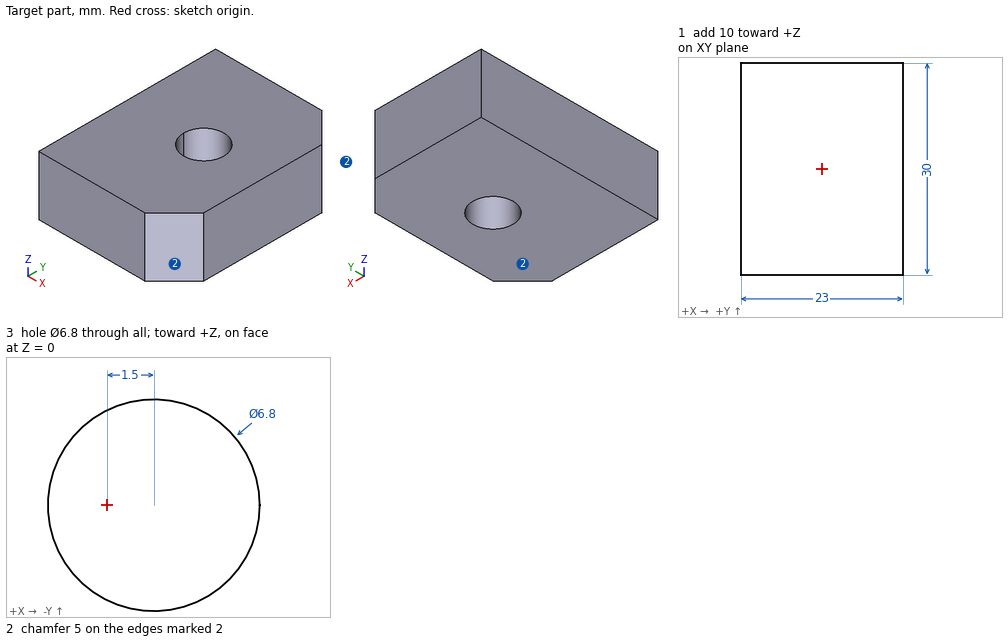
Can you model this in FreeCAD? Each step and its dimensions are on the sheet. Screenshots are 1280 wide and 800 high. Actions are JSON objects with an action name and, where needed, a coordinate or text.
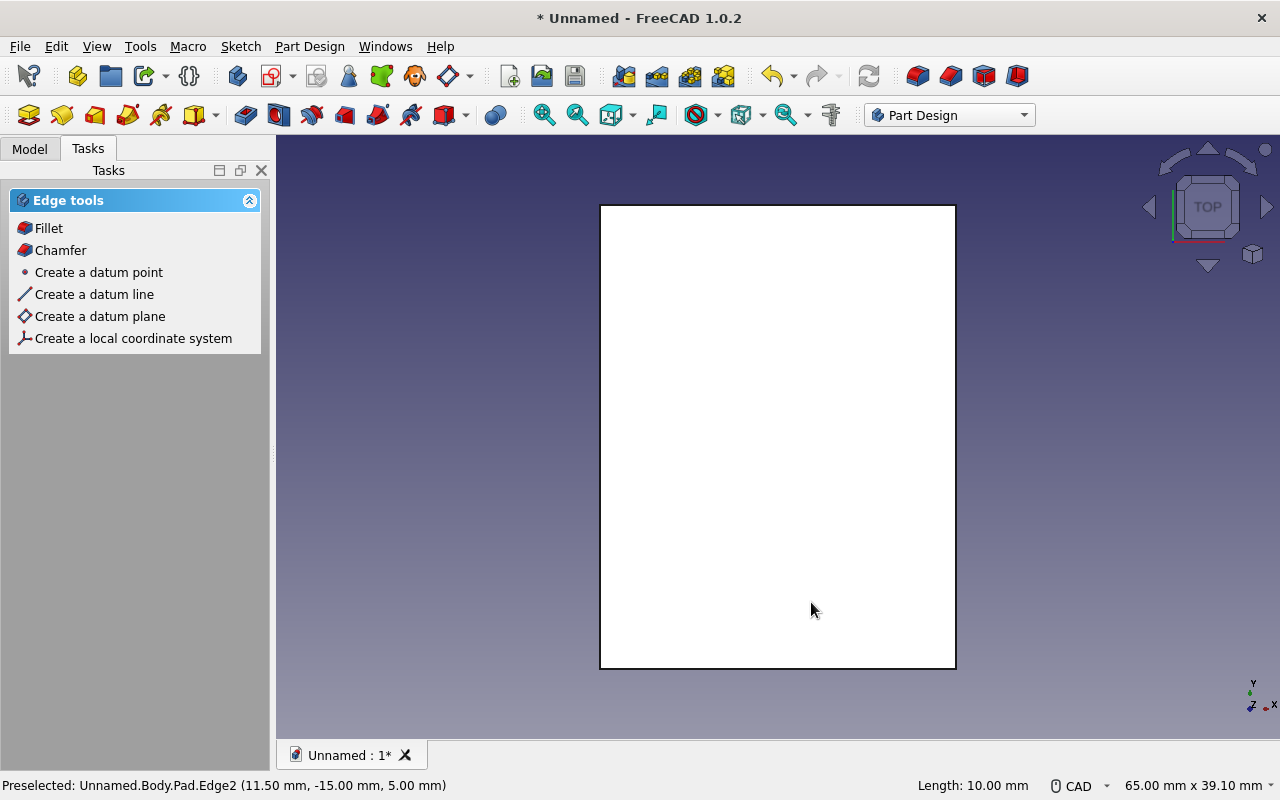
{"action": "key", "text": "1"}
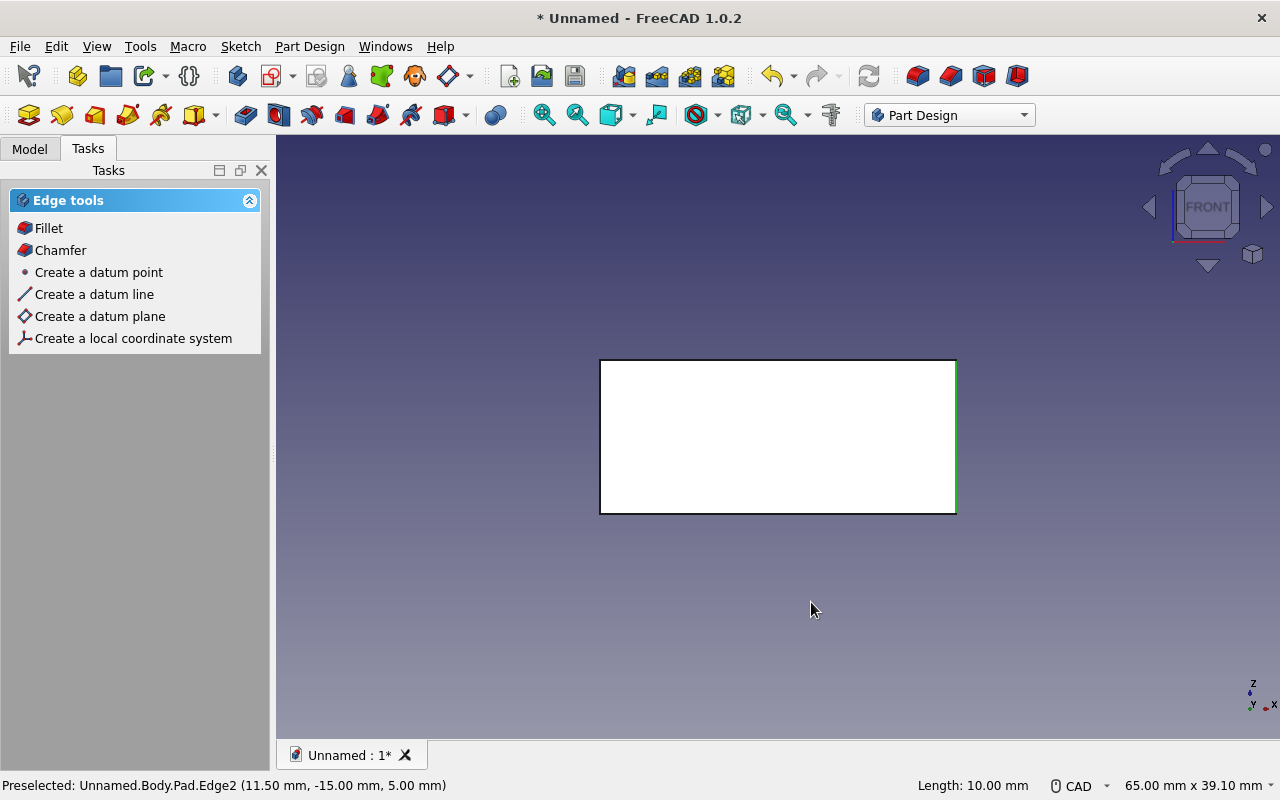
{"action": "key", "text": "v f"}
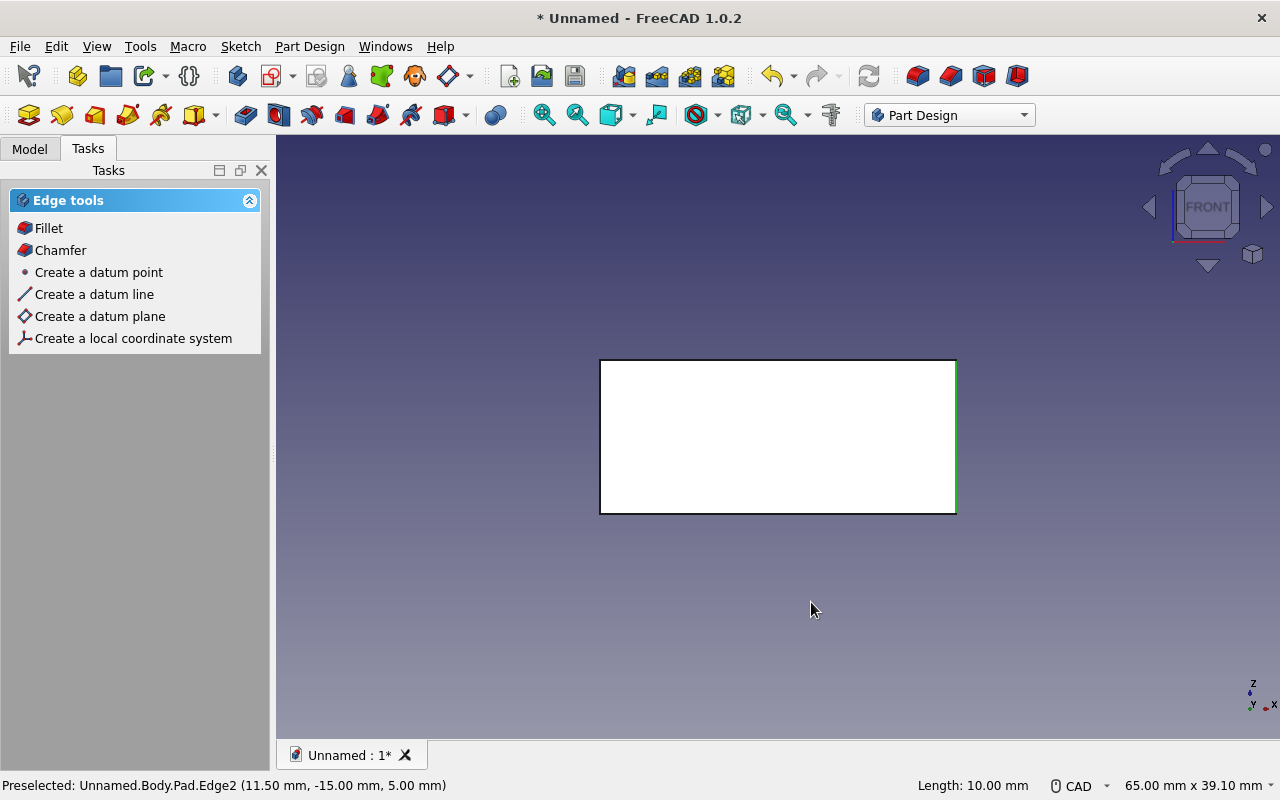
{"action": "key", "text": "3"}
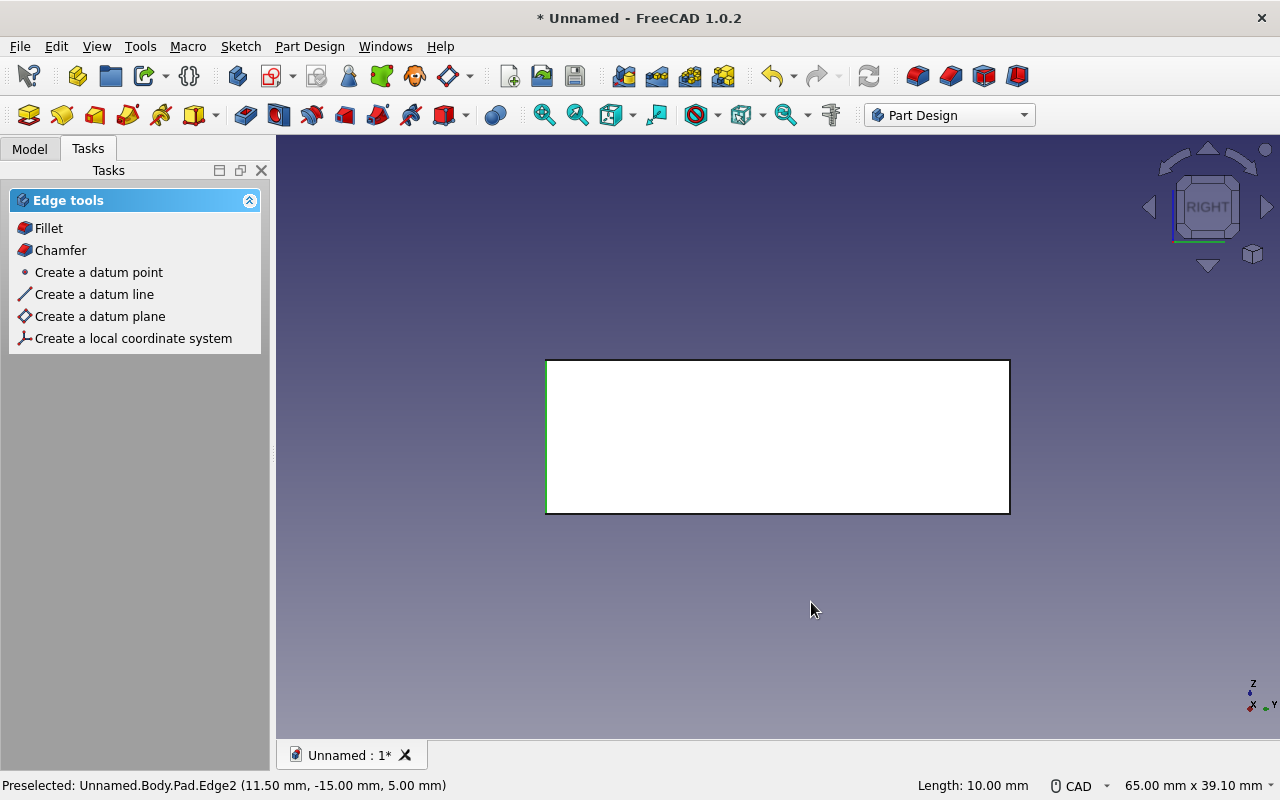
{"action": "left_click", "coordinate": [1010, 436], "text": "ctrl"}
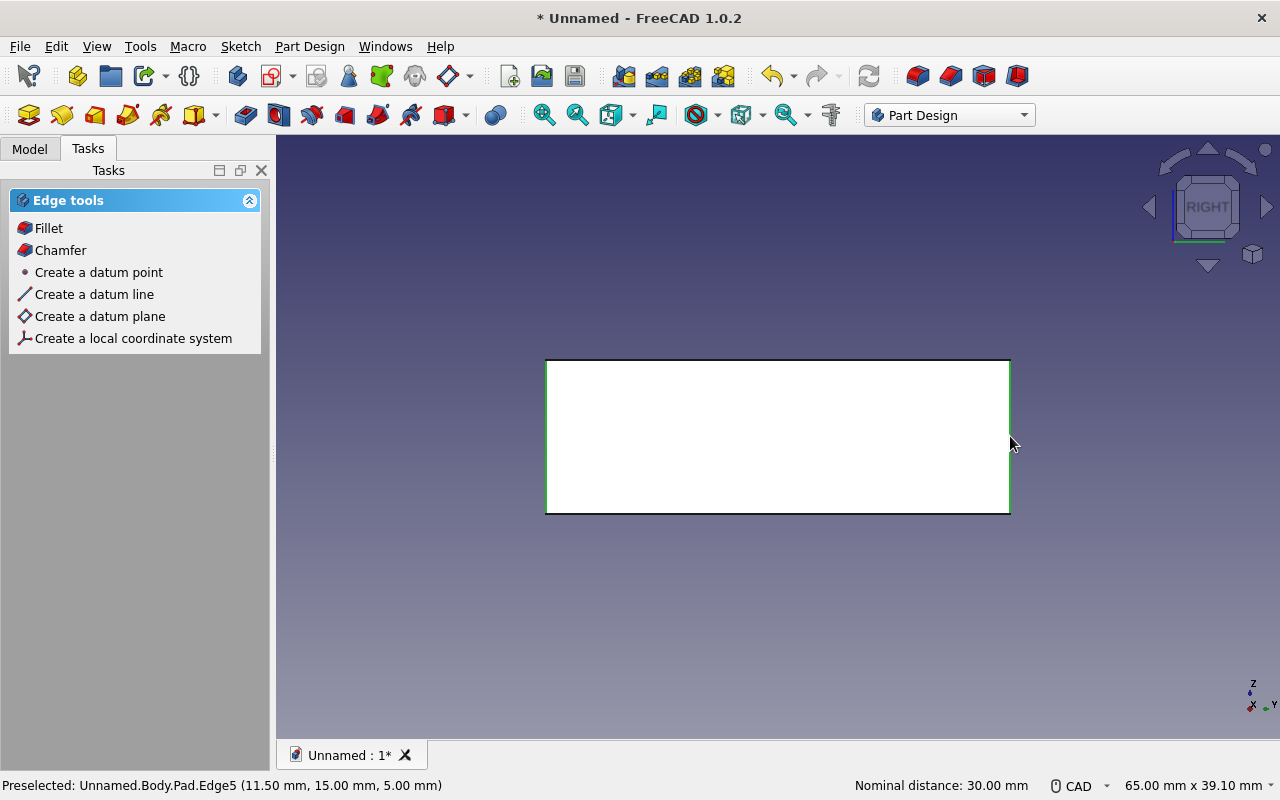
{"action": "left_click", "coordinate": [951, 76]}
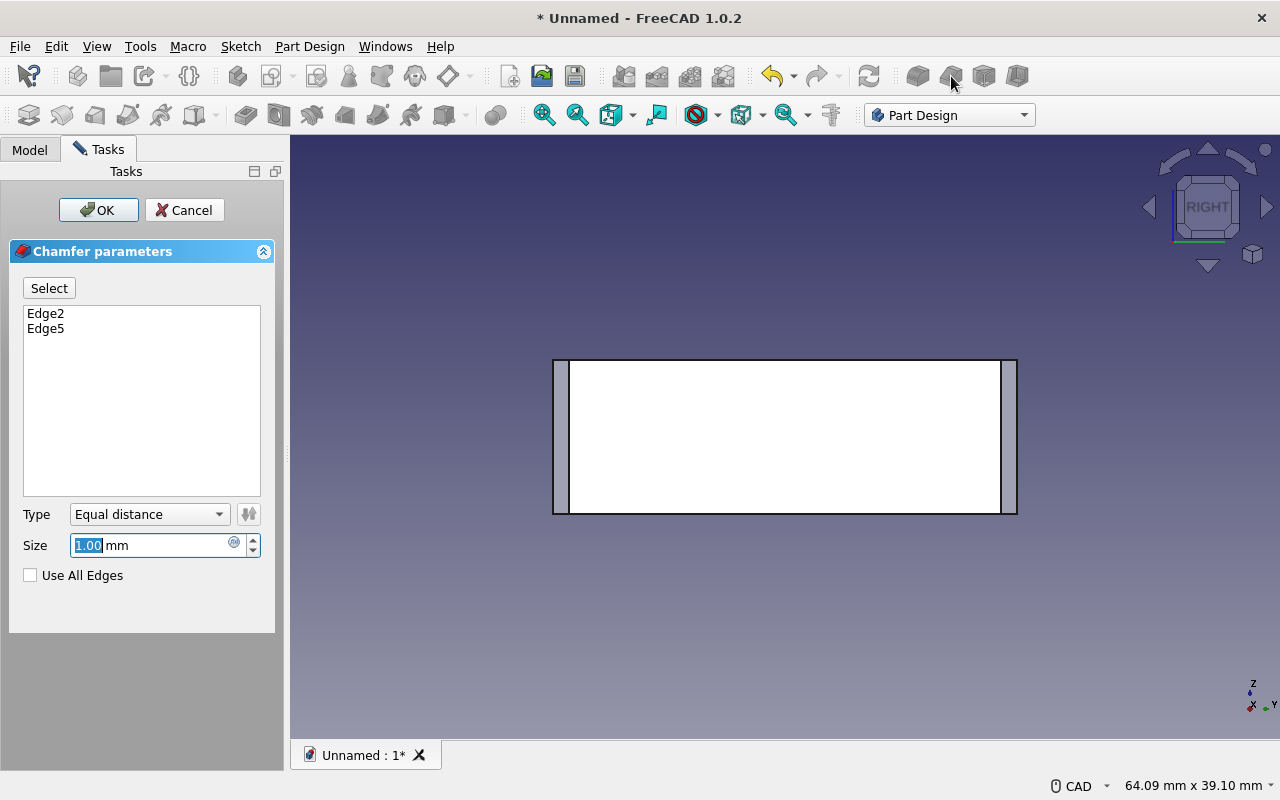
{"action": "type", "text": "5"}
{"action": "key", "text": "Tab"}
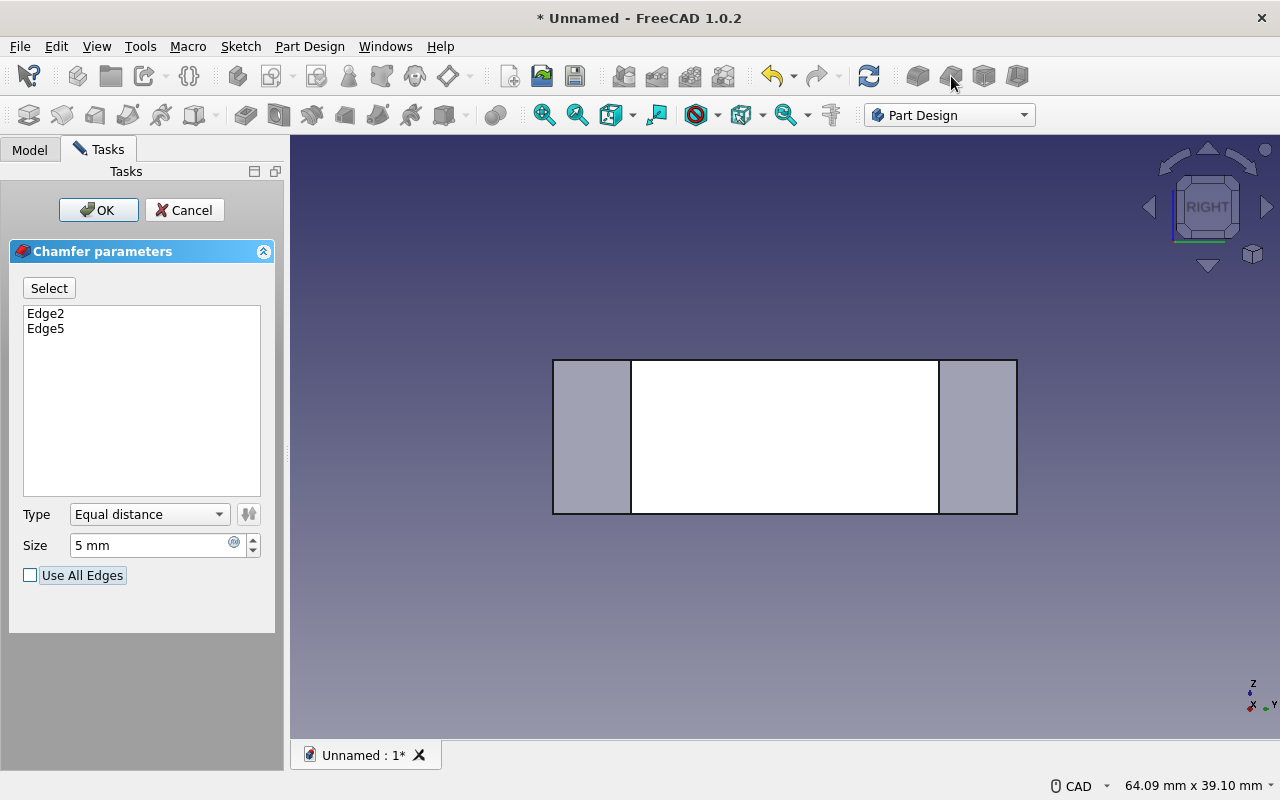
{"action": "left_click", "coordinate": [99, 210]}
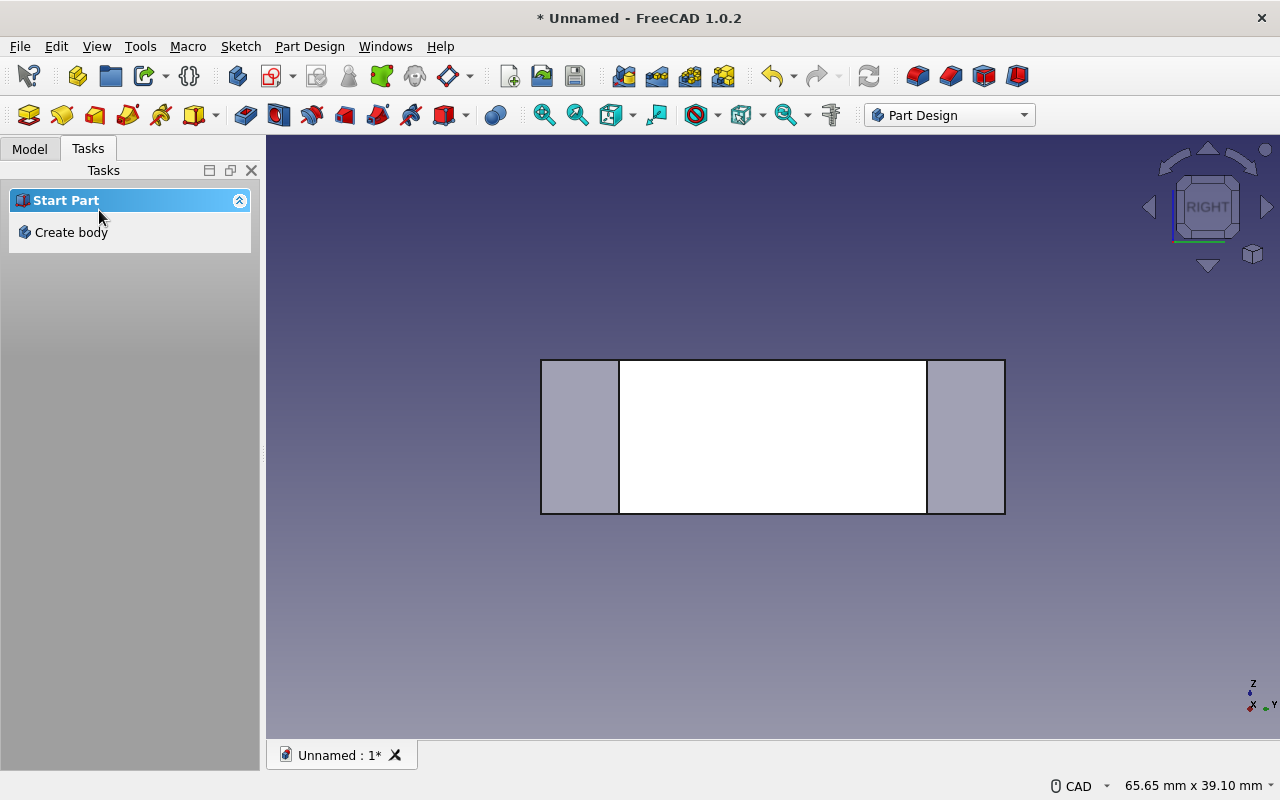
{"action": "key", "text": "5"}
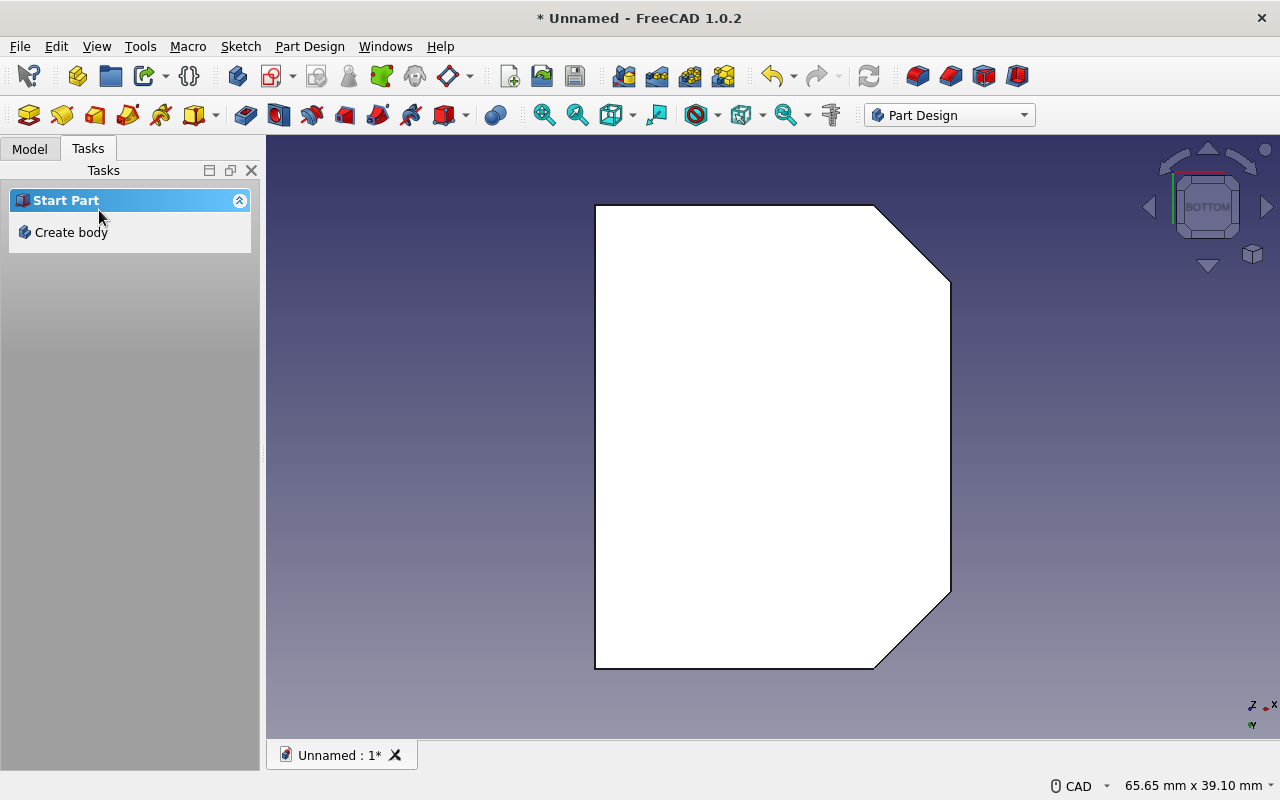
{"action": "left_click", "coordinate": [773, 436]}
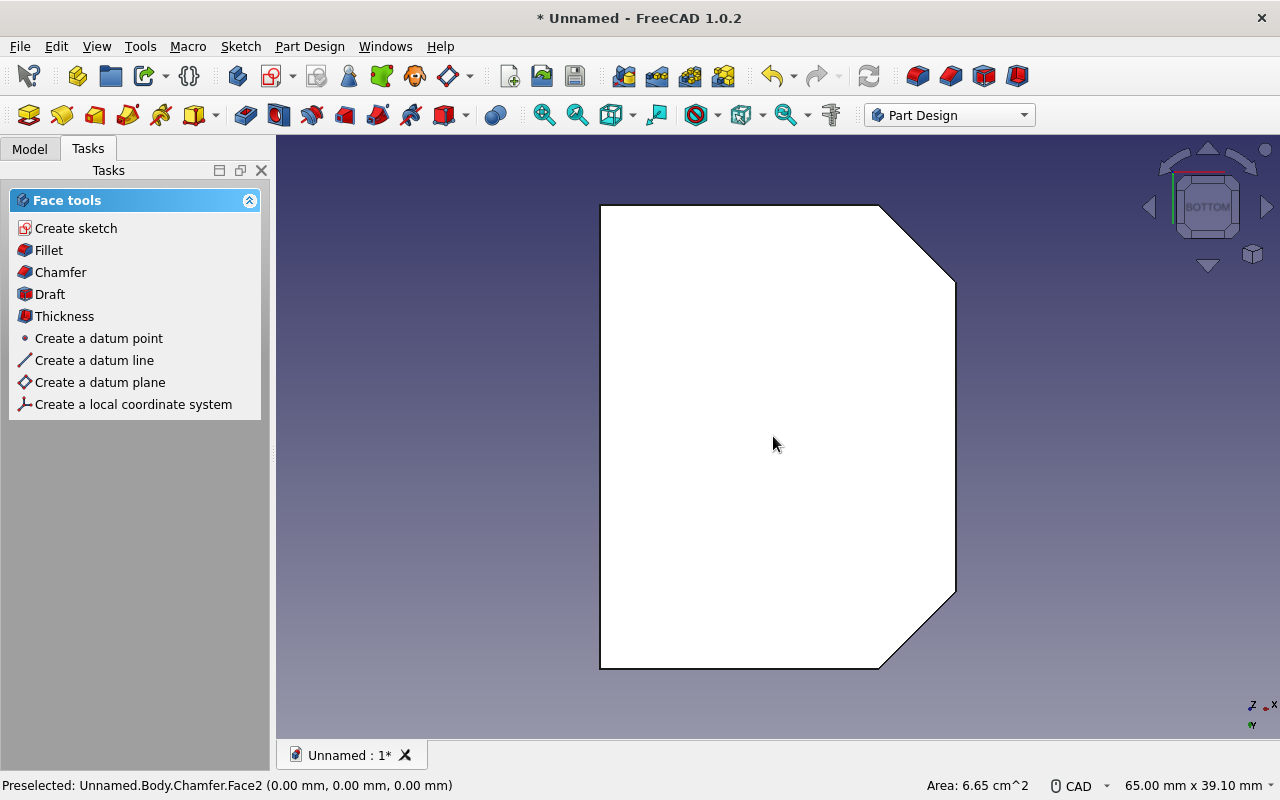
{"action": "left_click", "coordinate": [270, 76]}